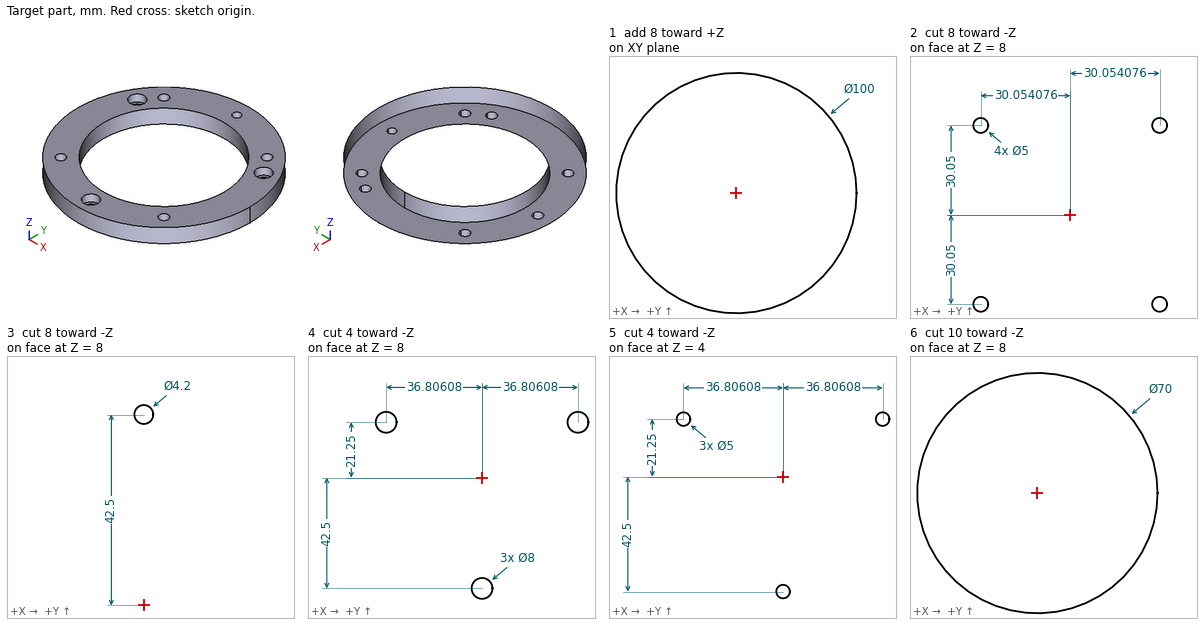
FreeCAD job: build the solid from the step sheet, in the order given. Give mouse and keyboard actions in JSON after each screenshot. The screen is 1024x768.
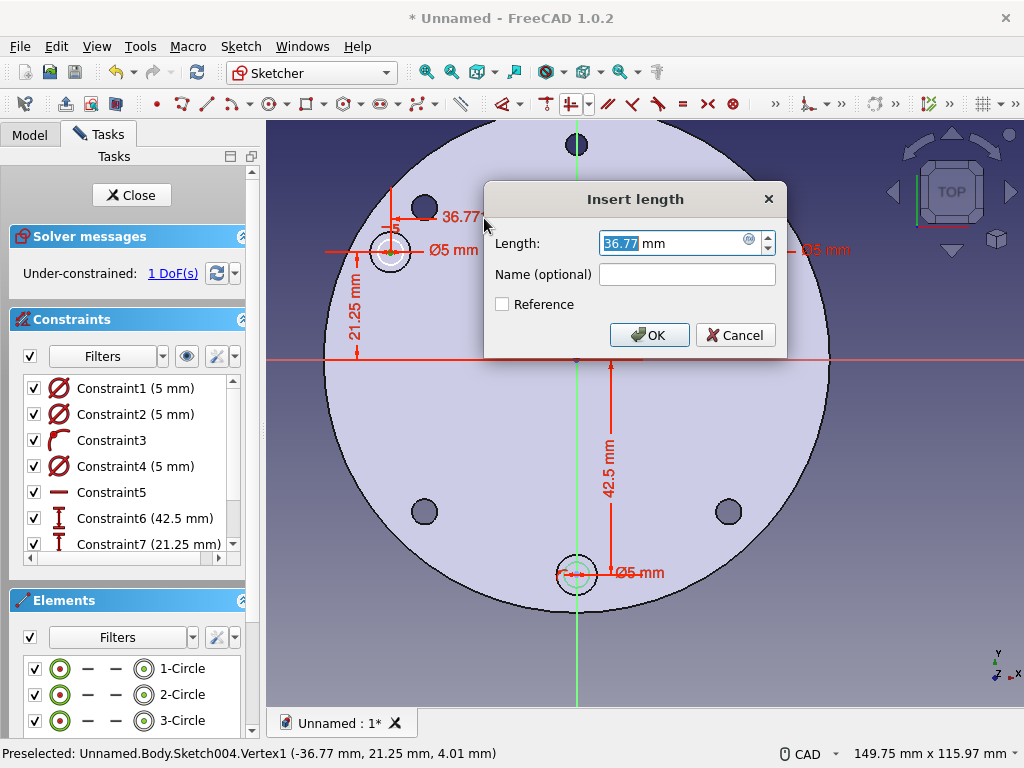
{"action": "type", "text": "36.80608"}
{"action": "key", "text": "Return"}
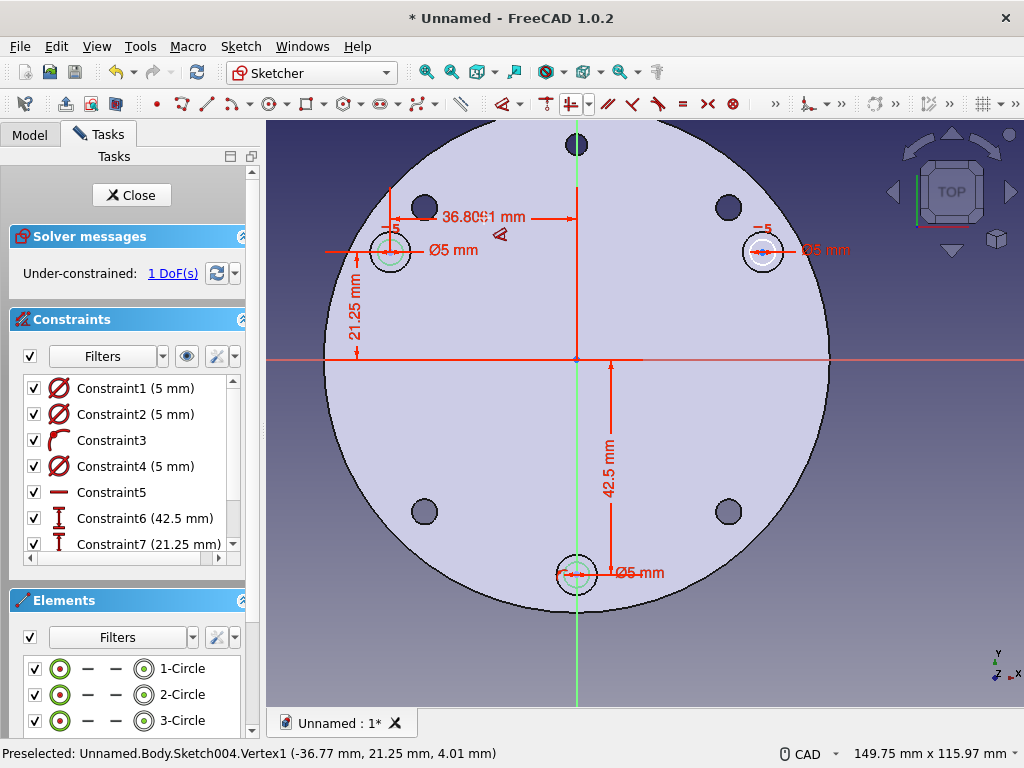
{"action": "left_click", "coordinate": [763, 252]}
{"action": "left_click", "coordinate": [670, 218]}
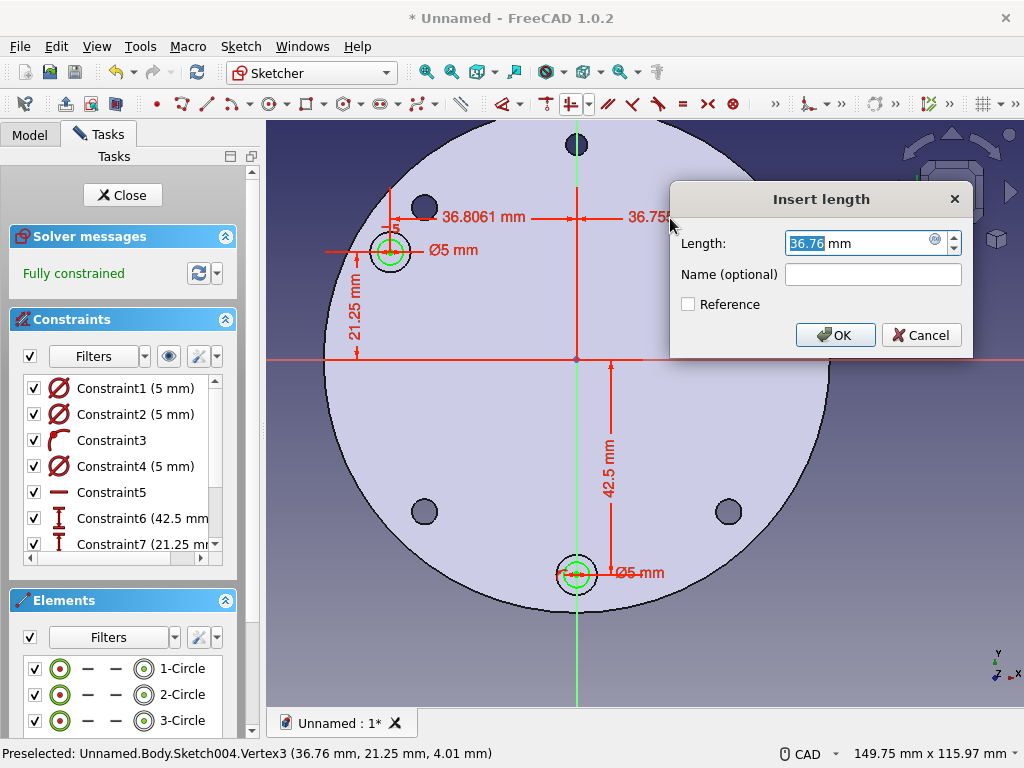
{"action": "type", "text": "36.80608"}
{"action": "key", "text": "Return"}
{"action": "key", "text": "Escape"}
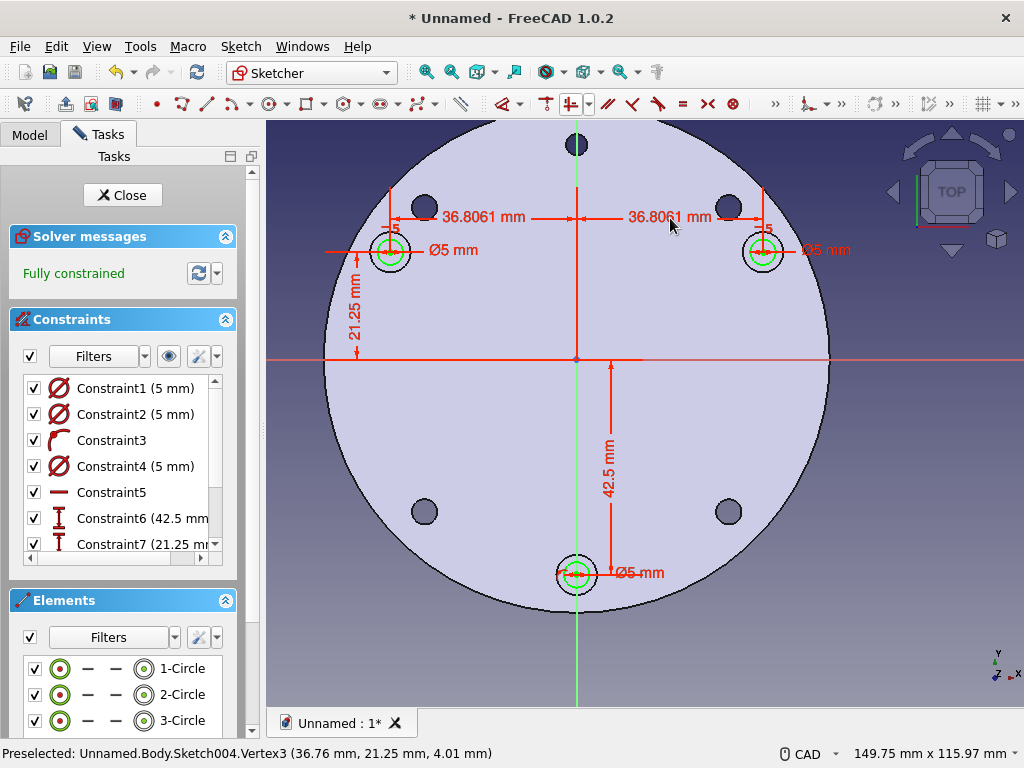
{"action": "left_click", "coordinate": [123, 195]}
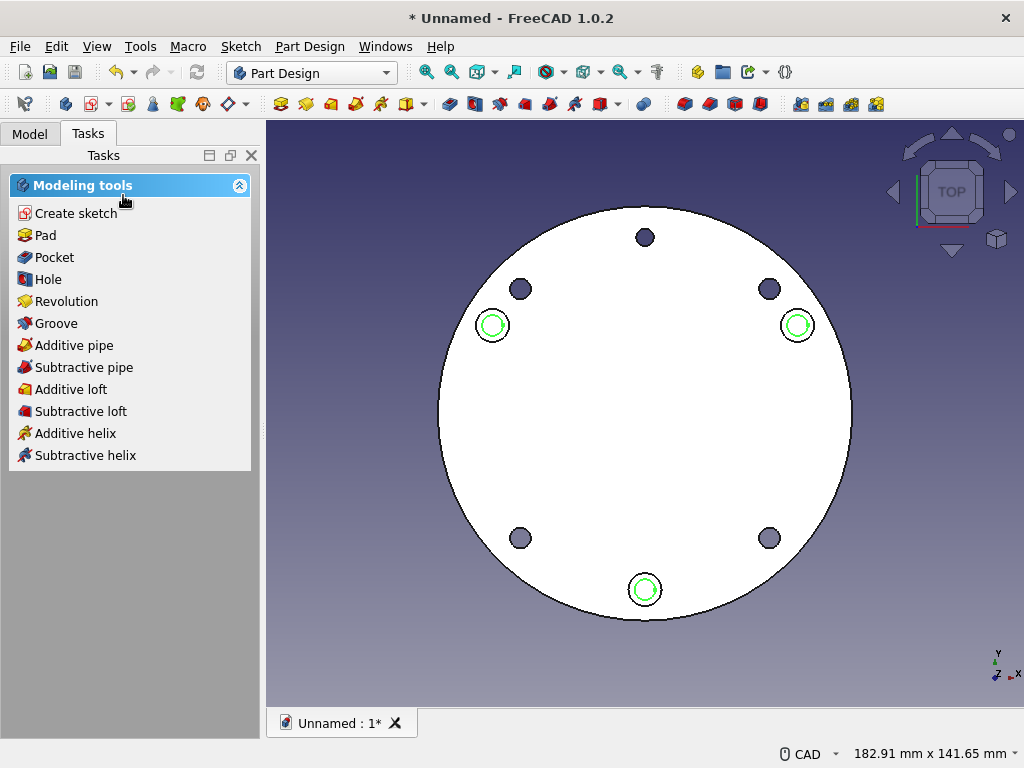
{"action": "left_click", "coordinate": [450, 104]}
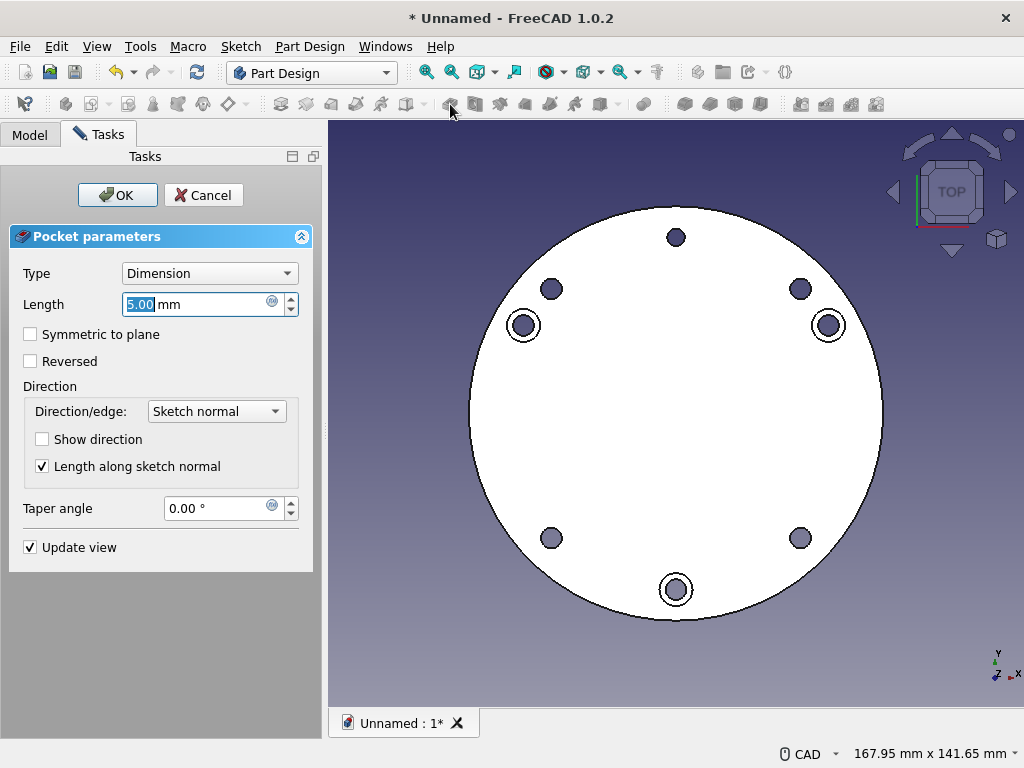
{"action": "type", "text": "4"}
{"action": "key", "text": "Tab"}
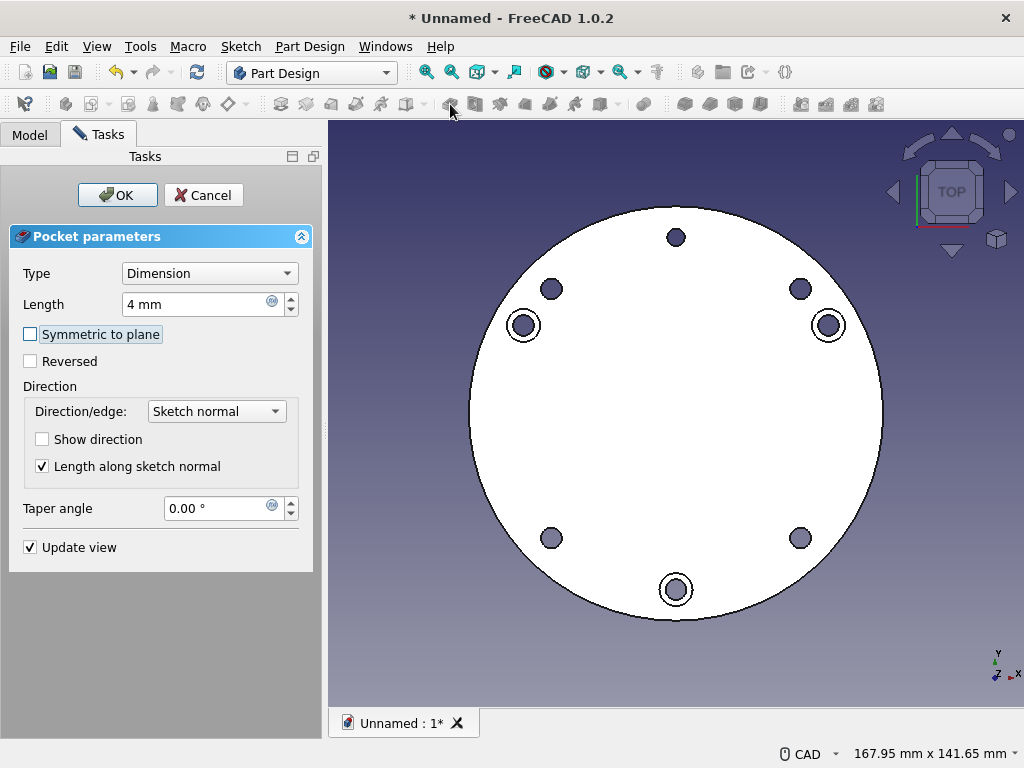
{"action": "left_click", "coordinate": [118, 195]}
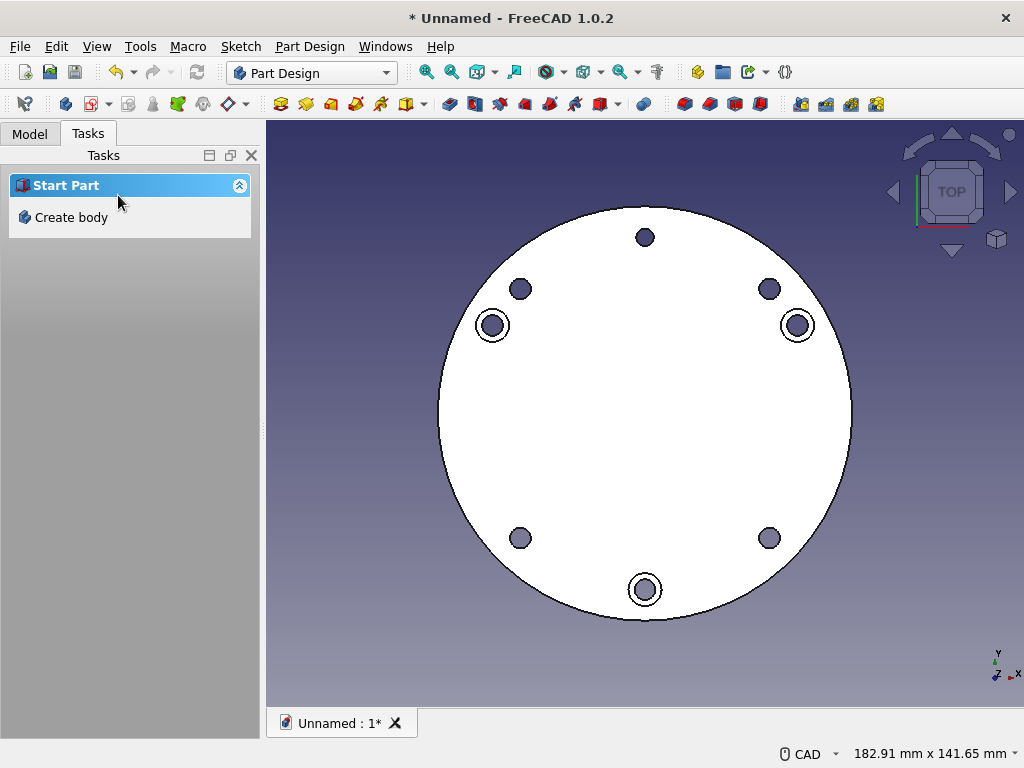
{"action": "left_click", "coordinate": [645, 413]}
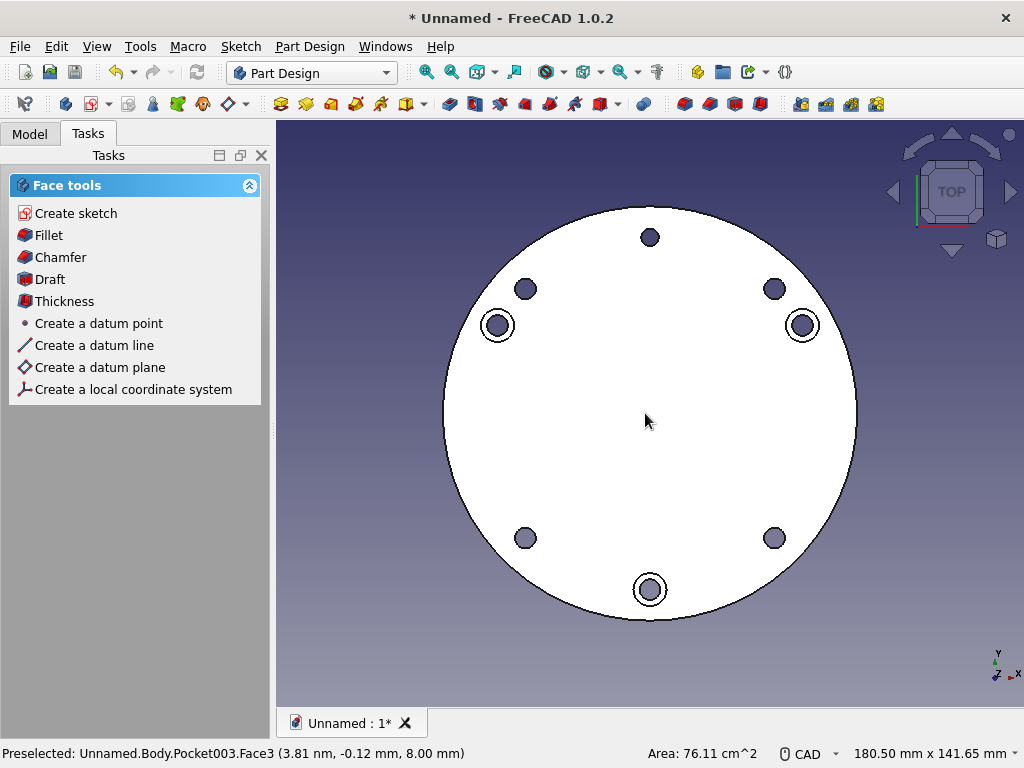
{"action": "left_click", "coordinate": [90, 104]}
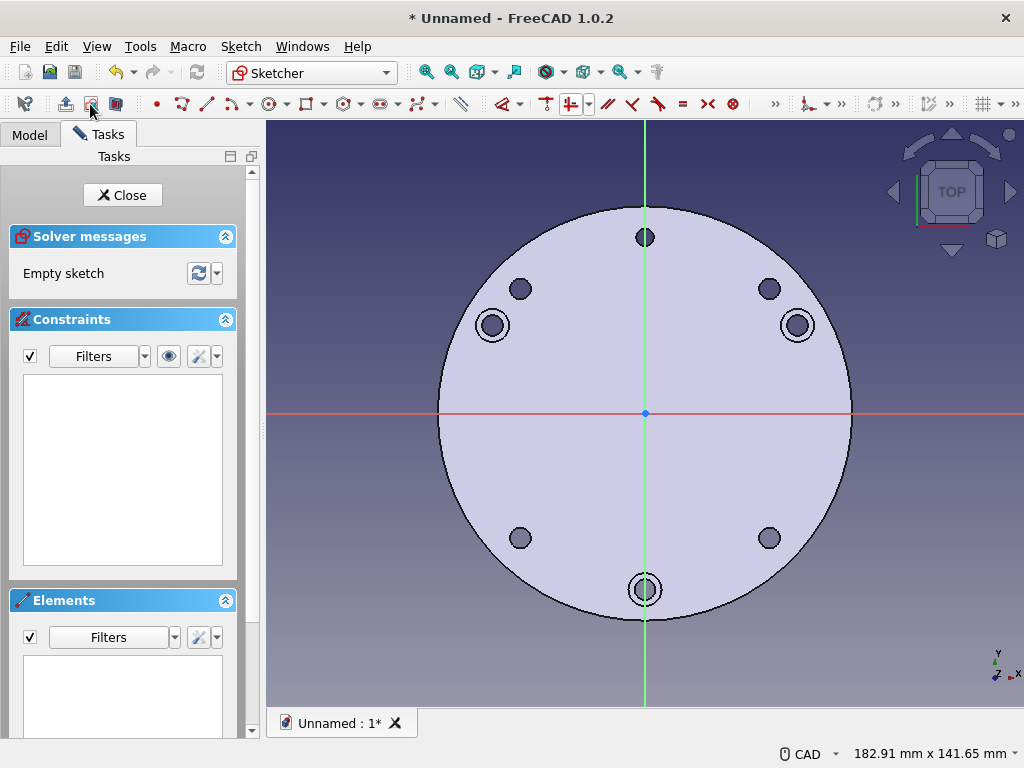
{"action": "left_click", "coordinate": [268, 104]}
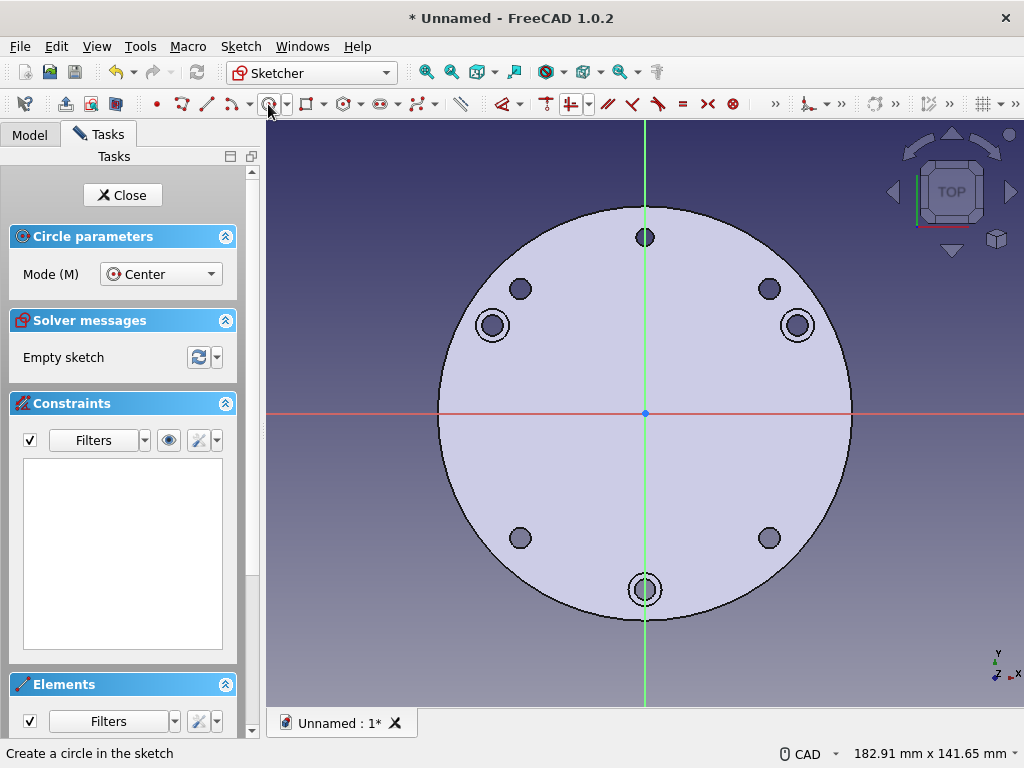
{"action": "left_click", "coordinate": [645, 414]}
{"action": "mouse_move", "coordinate": [748, 311]}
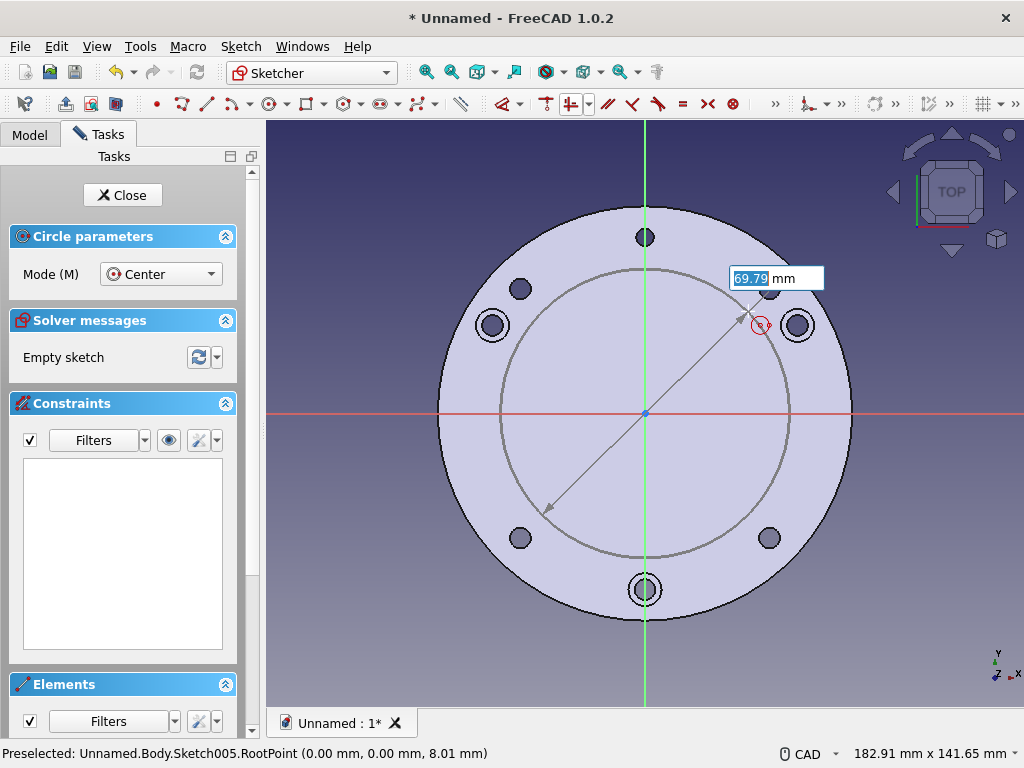
{"action": "type", "text": "70"}
{"action": "key", "text": "Return"}
{"action": "key", "text": "Escape"}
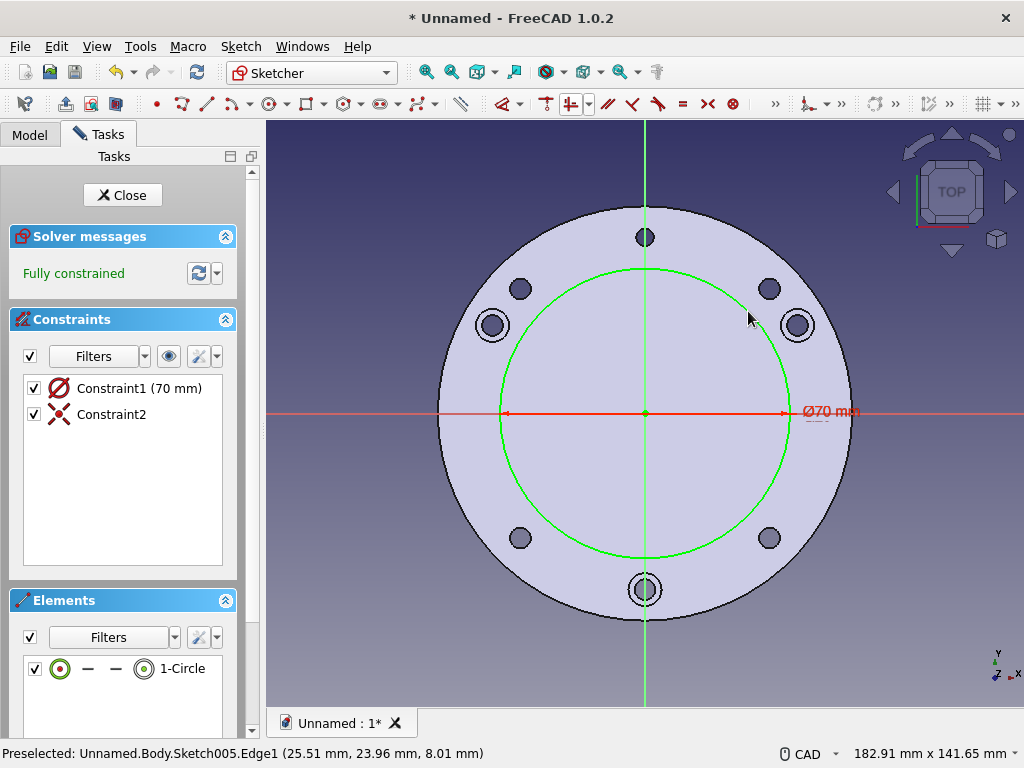
{"action": "left_click", "coordinate": [123, 195]}